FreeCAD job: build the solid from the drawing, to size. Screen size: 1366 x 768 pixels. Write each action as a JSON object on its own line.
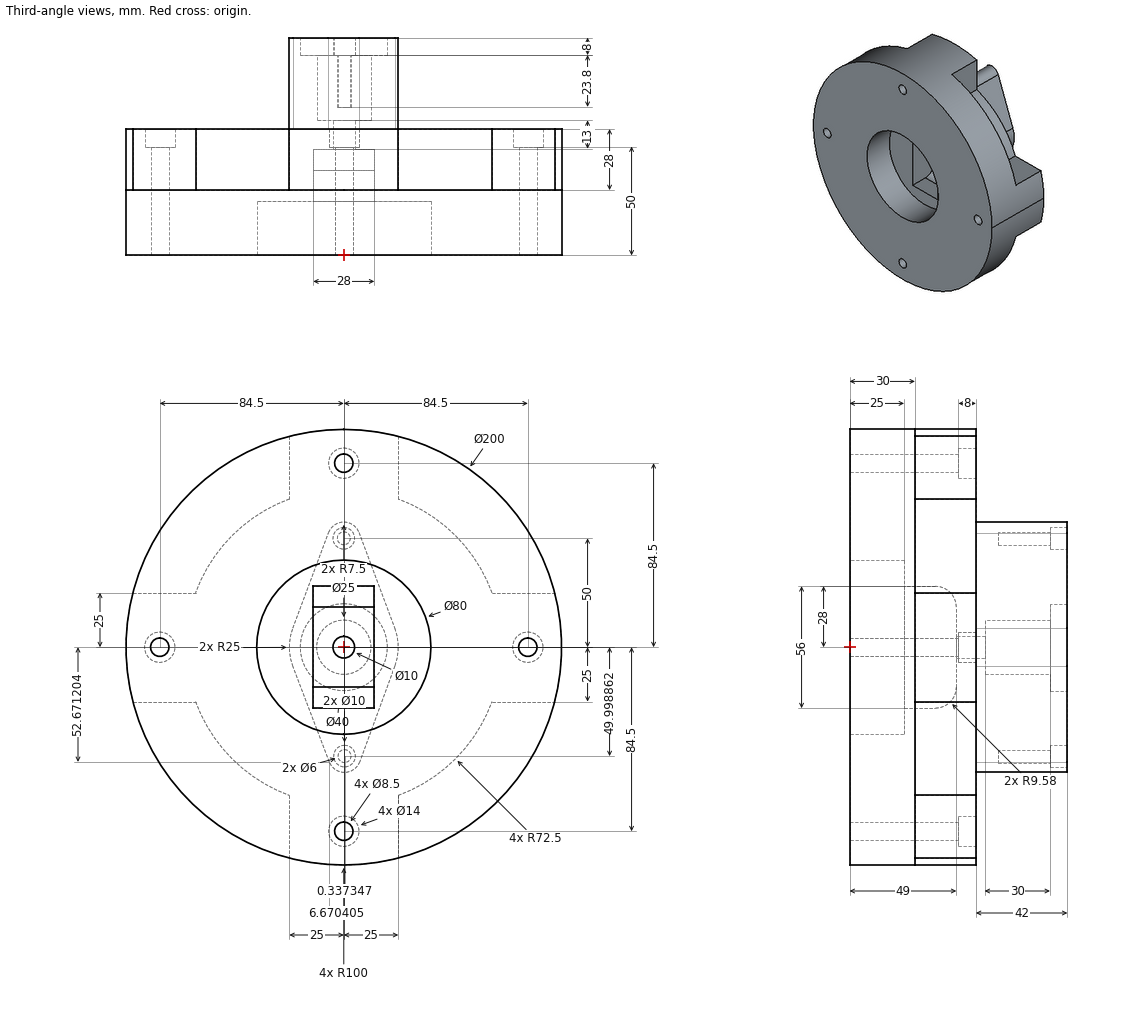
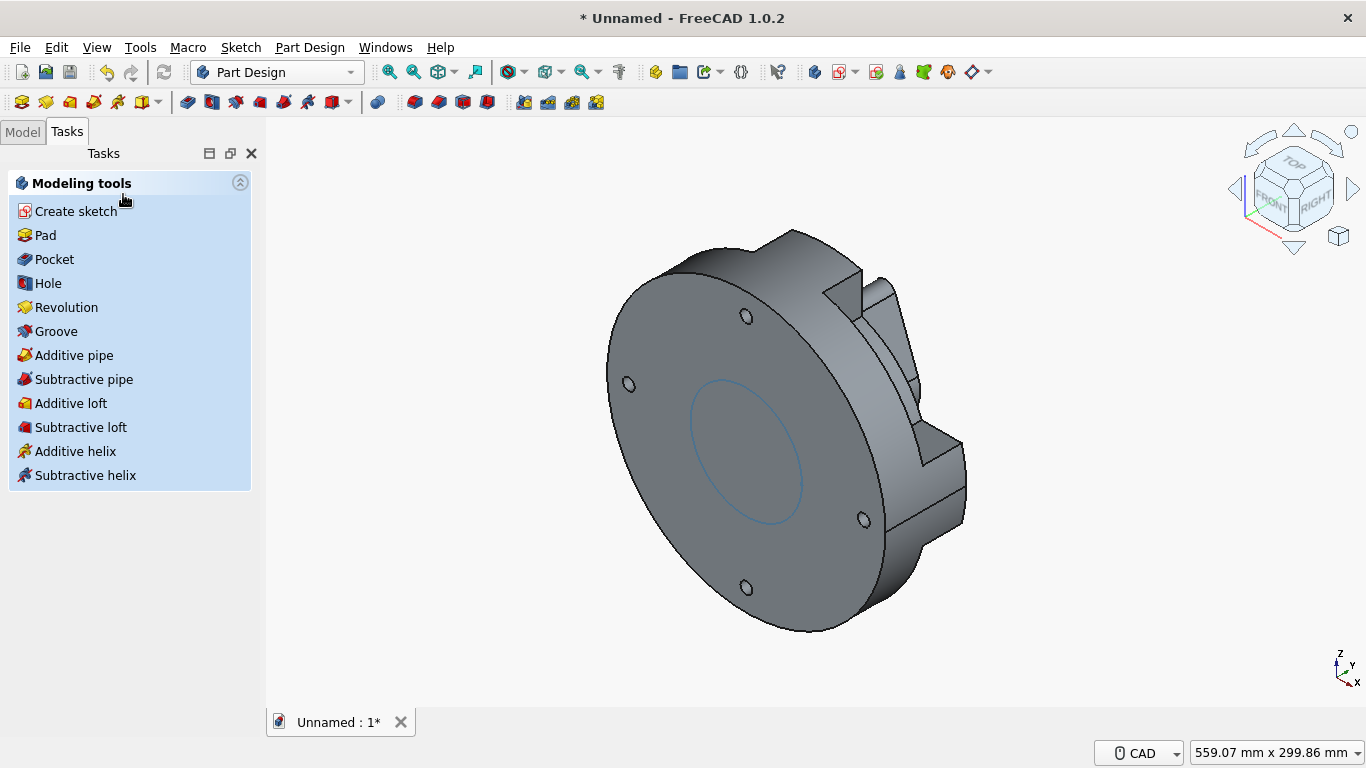
{"action": "left_click", "coordinate": [188, 102]}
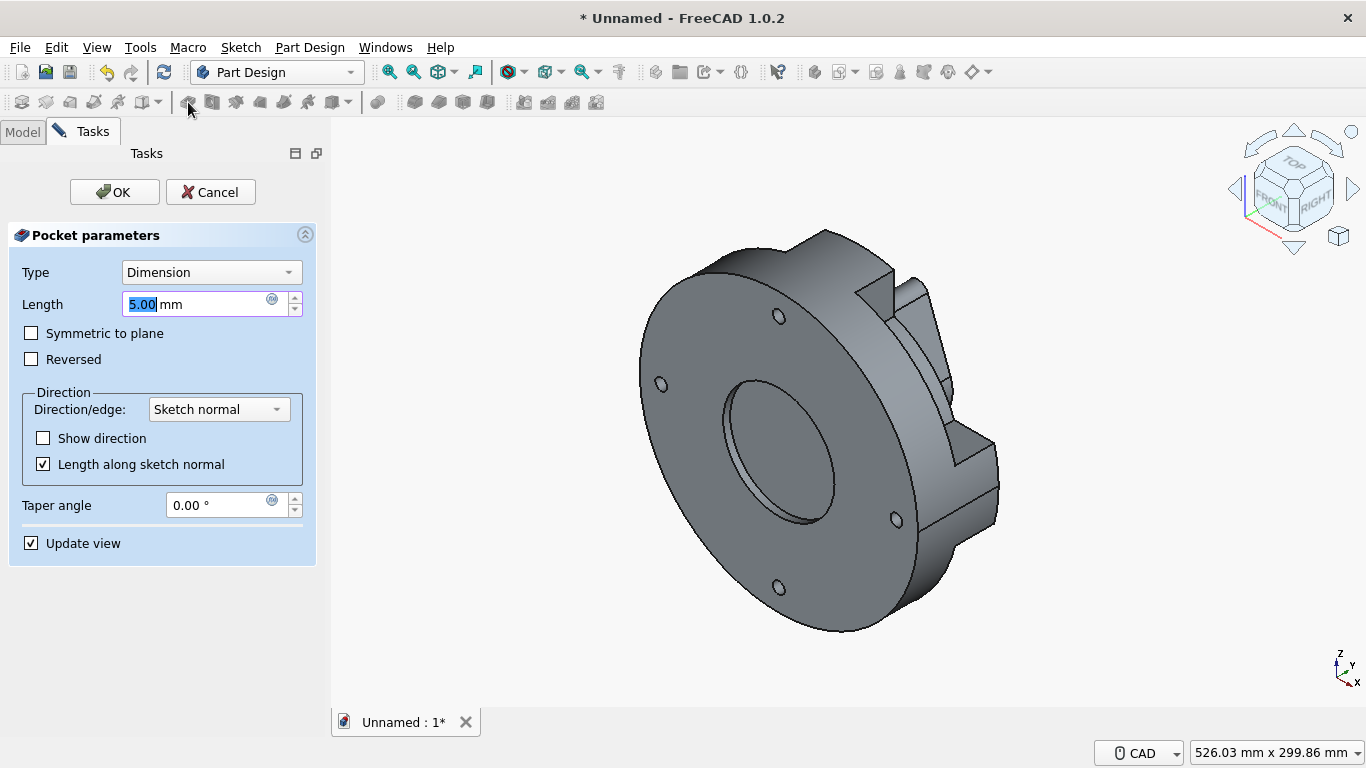
{"action": "type", "text": "25"}
{"action": "key", "text": "Tab"}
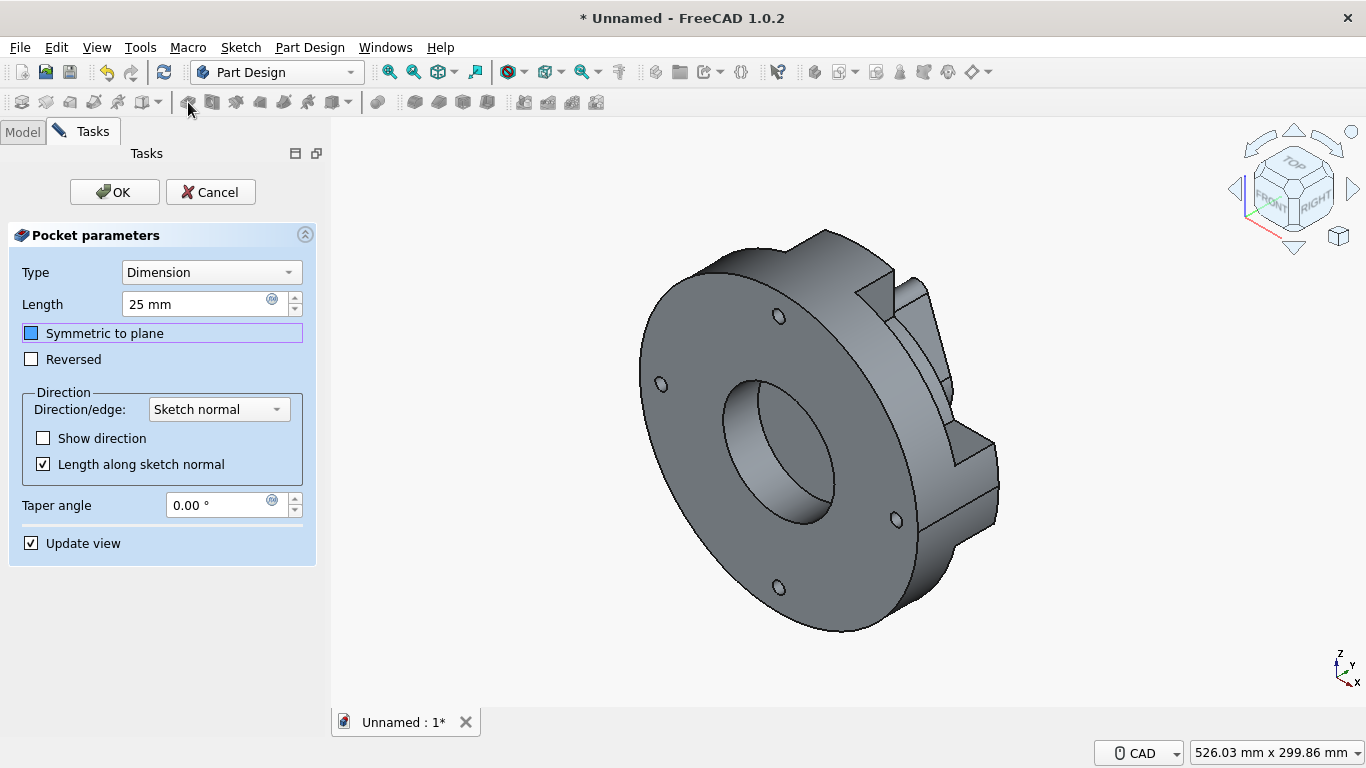
{"action": "left_click", "coordinate": [115, 192]}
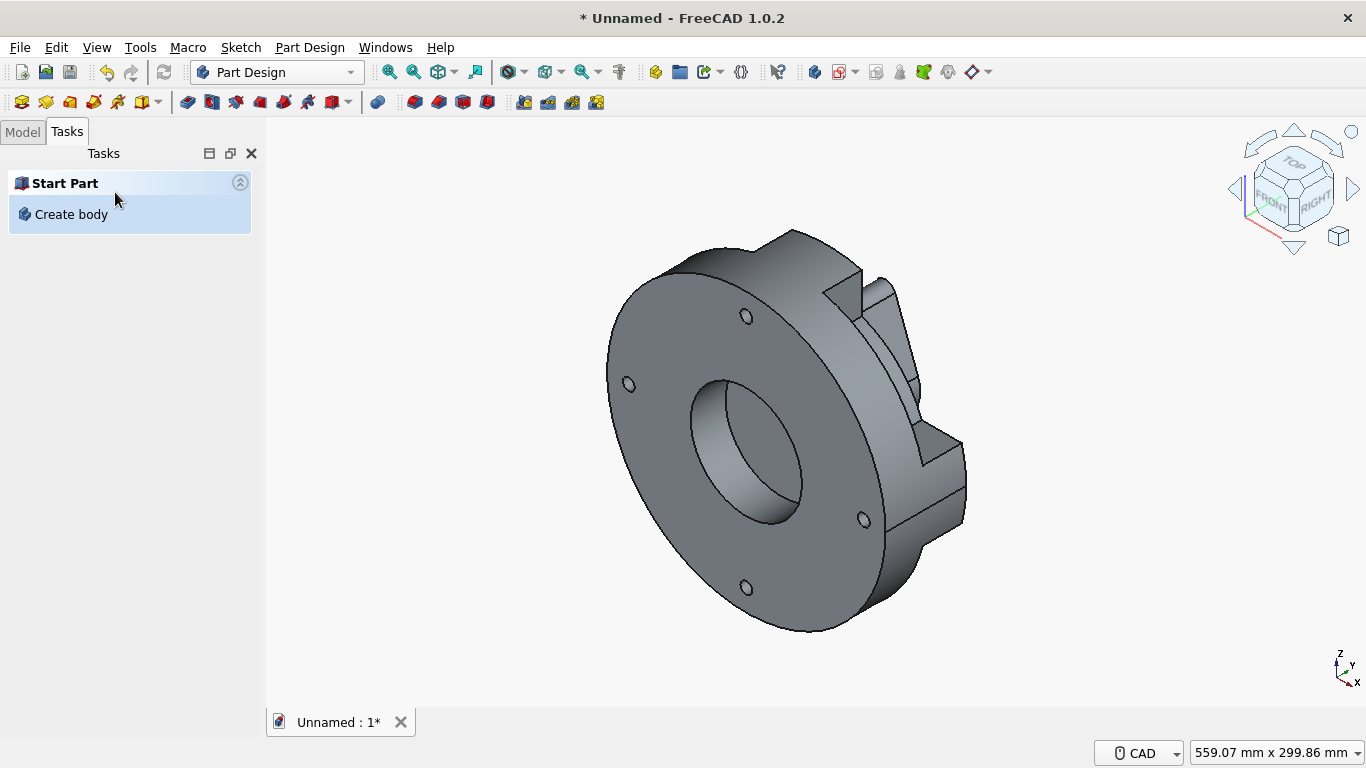
{"action": "left_click", "coordinate": [840, 72]}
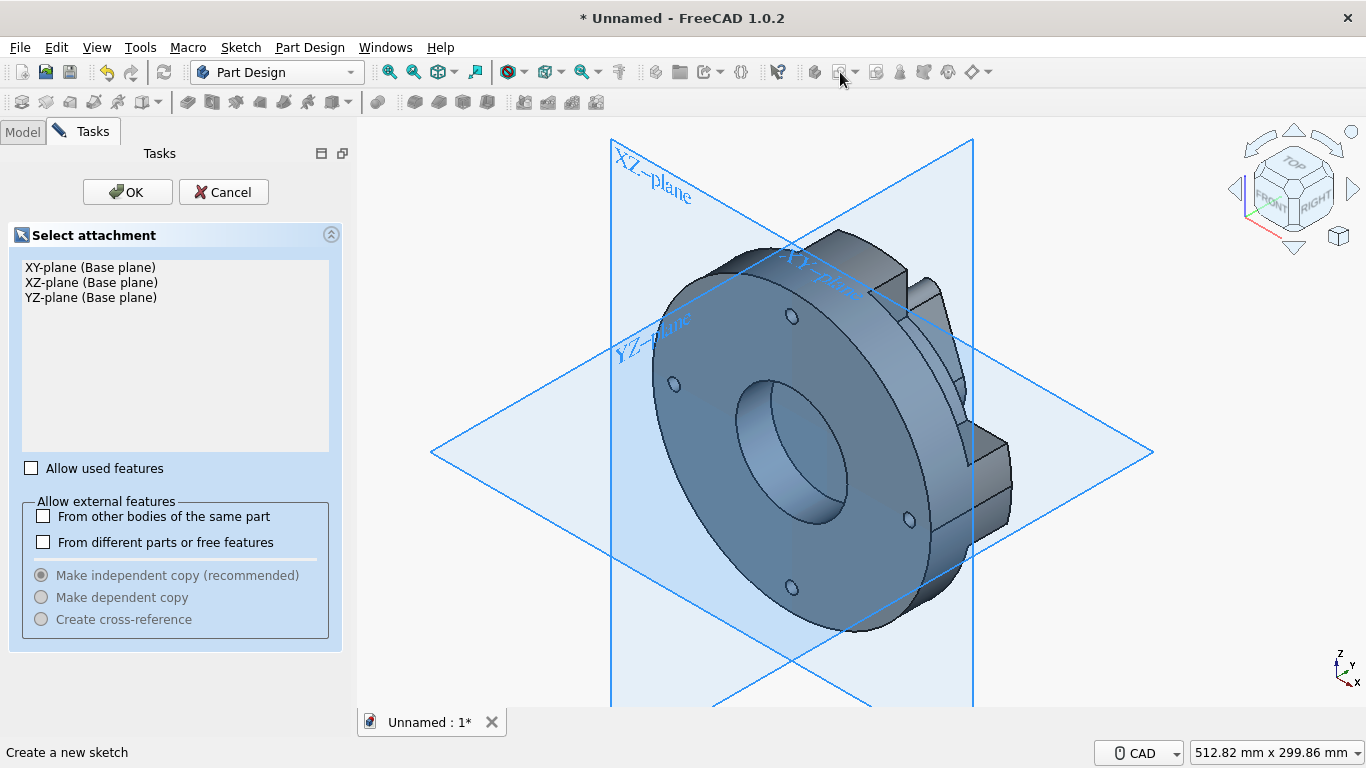
{"action": "left_click", "coordinate": [82, 298]}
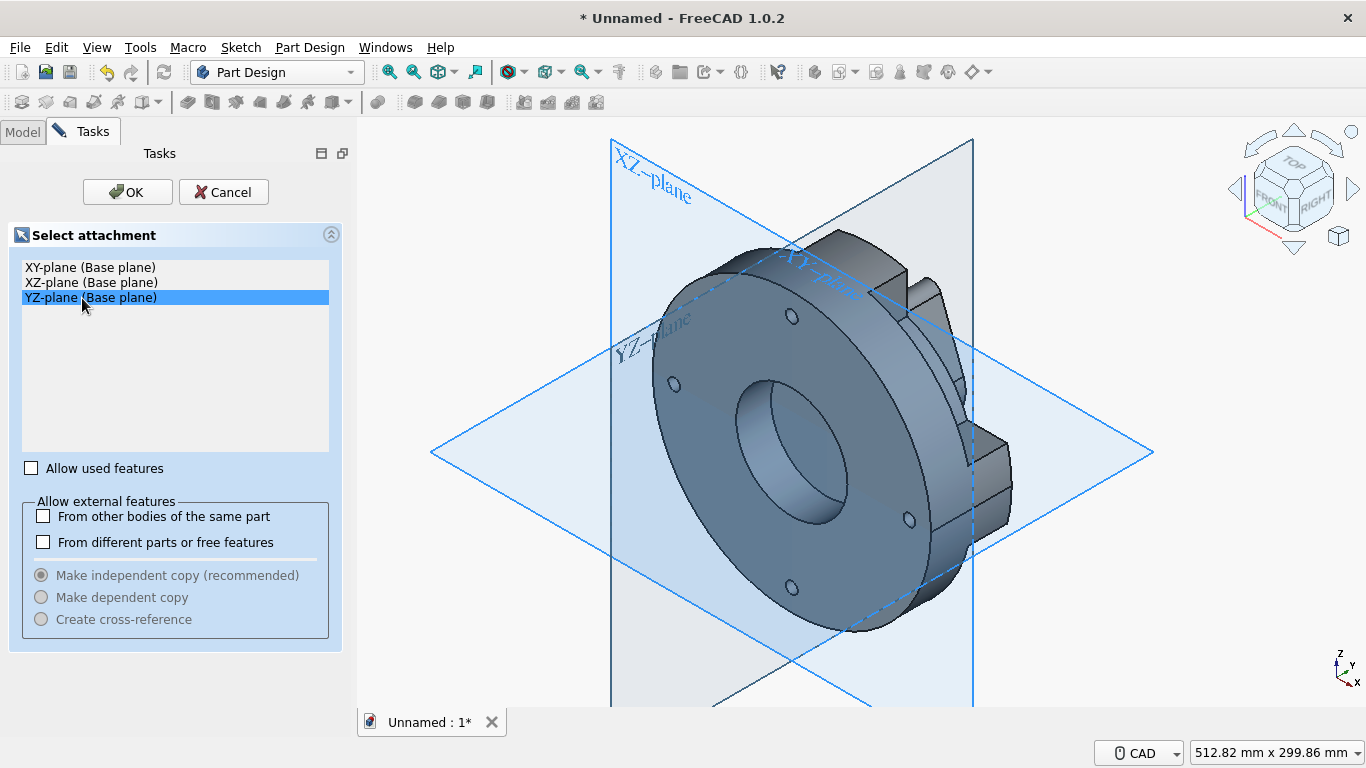
{"action": "left_click", "coordinate": [128, 192]}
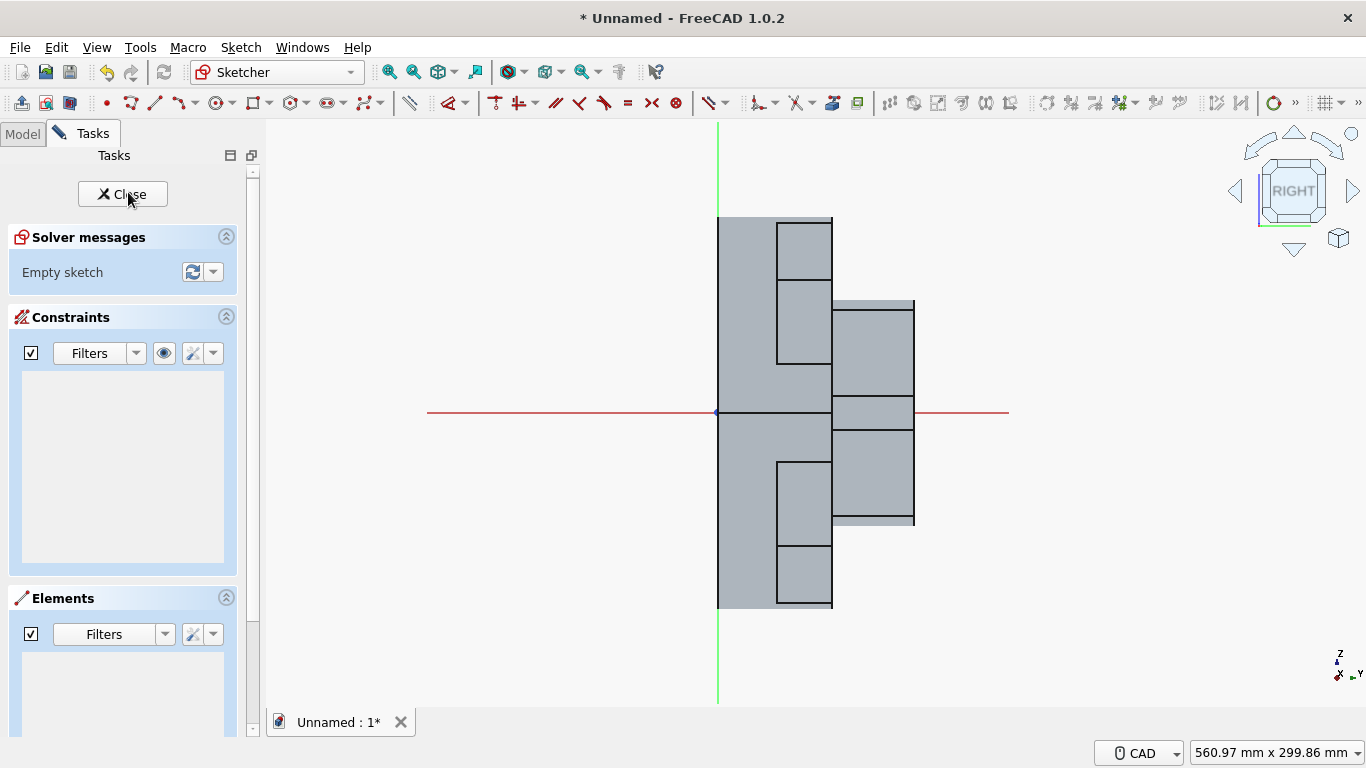
{"action": "key", "text": "q s"}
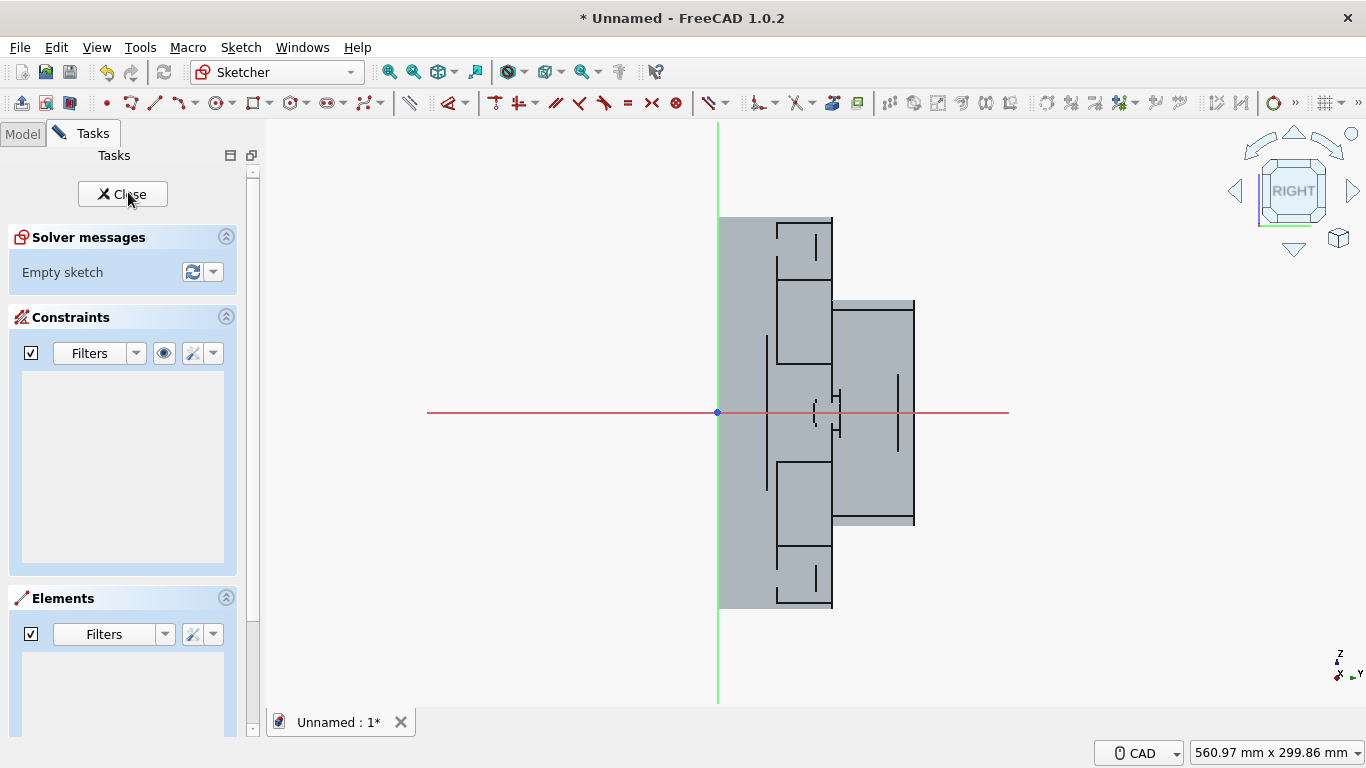
{"action": "scroll", "coordinate": [774, 413], "scroll_direction": "up", "scroll_amount": 6}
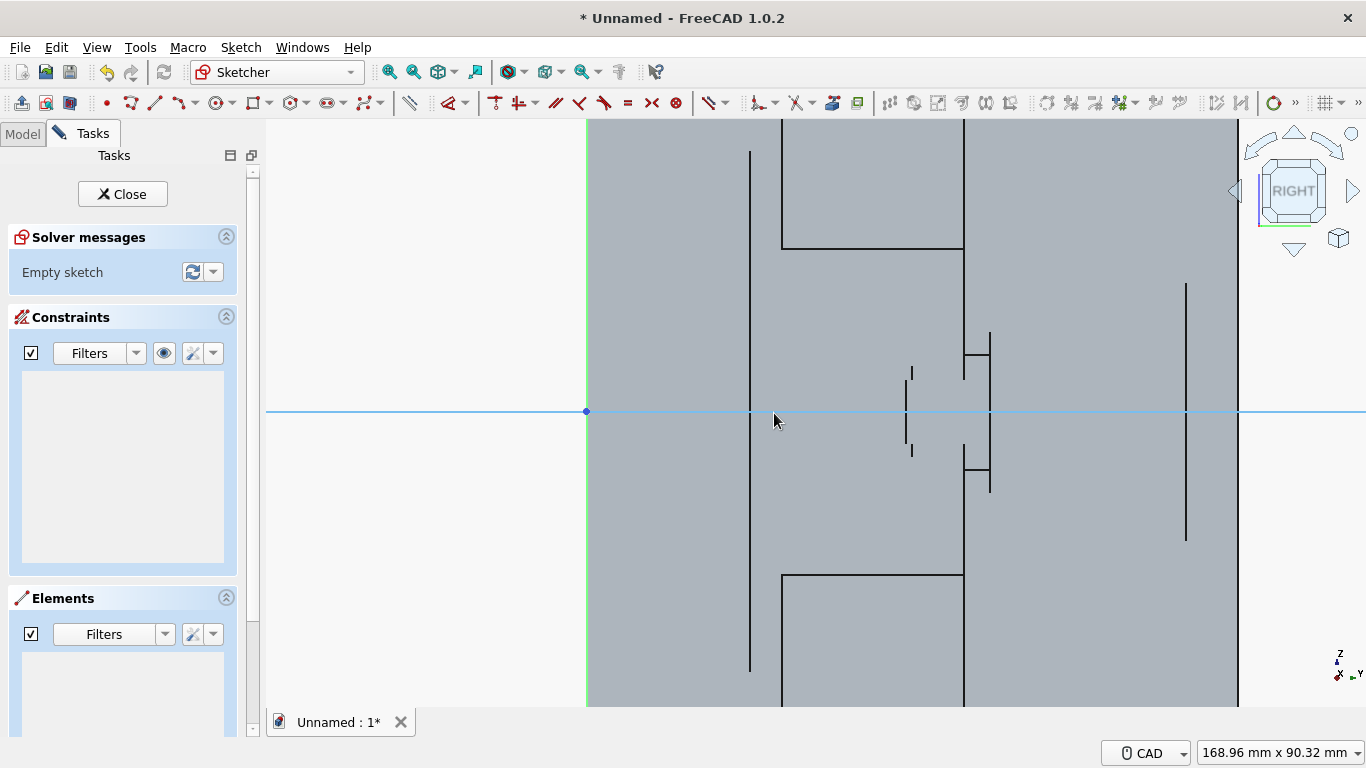
{"action": "left_click", "coordinate": [156, 104]}